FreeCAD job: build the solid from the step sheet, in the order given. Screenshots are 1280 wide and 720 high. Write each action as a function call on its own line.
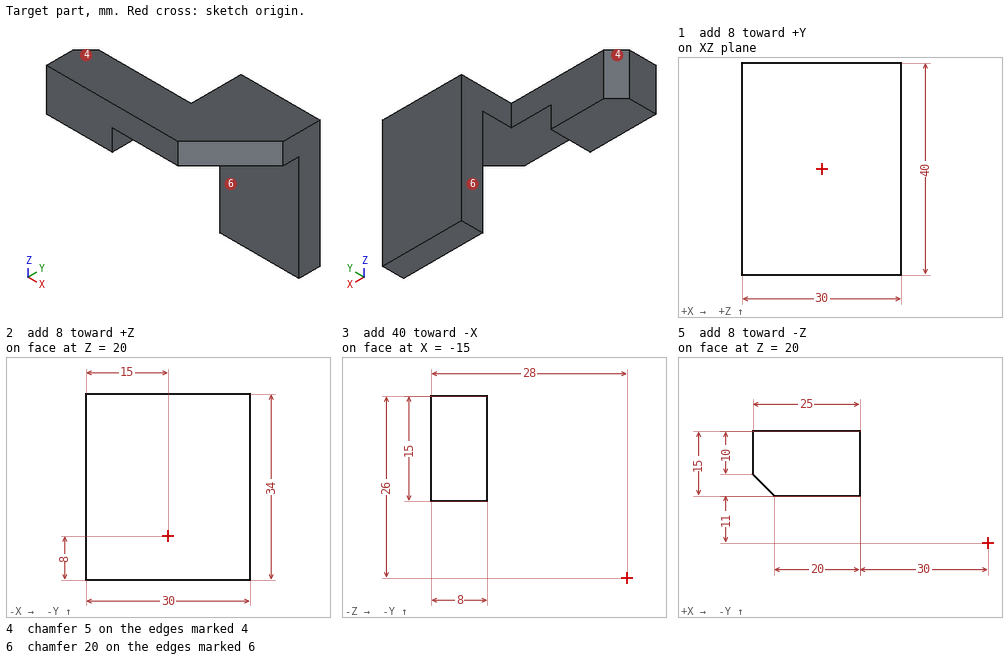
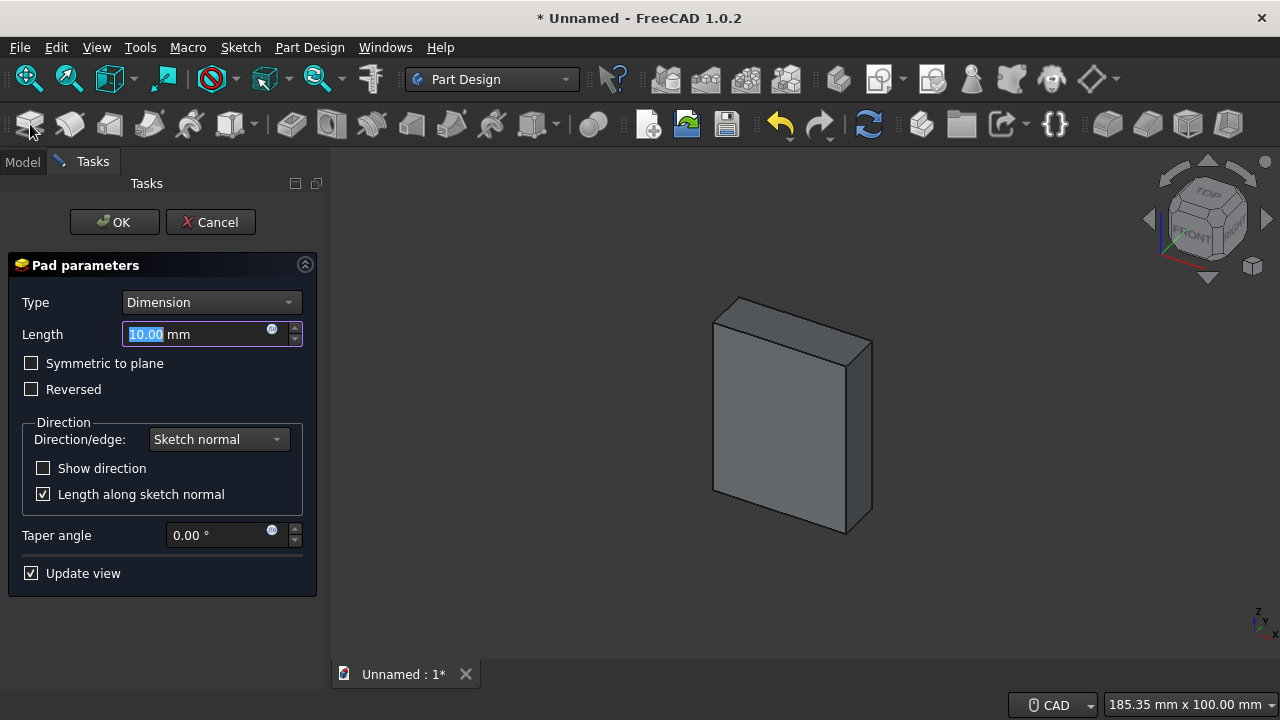
text(8)
key(Tab)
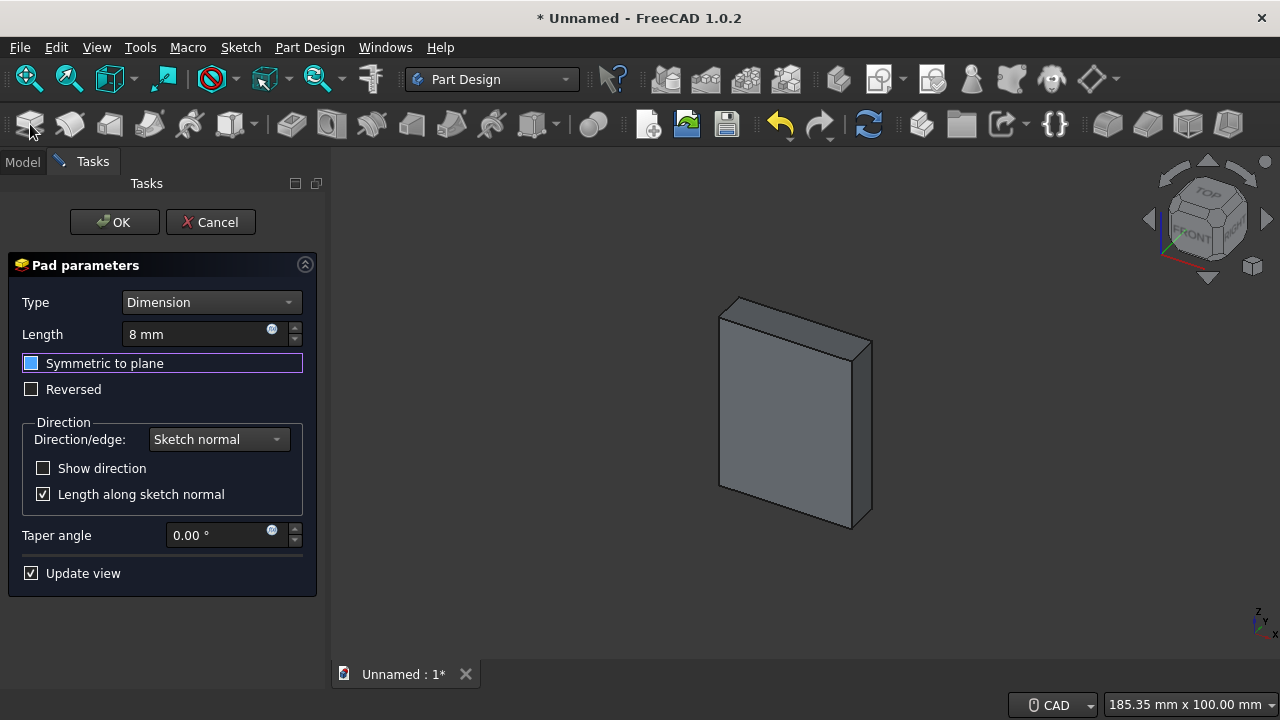
click(30, 389)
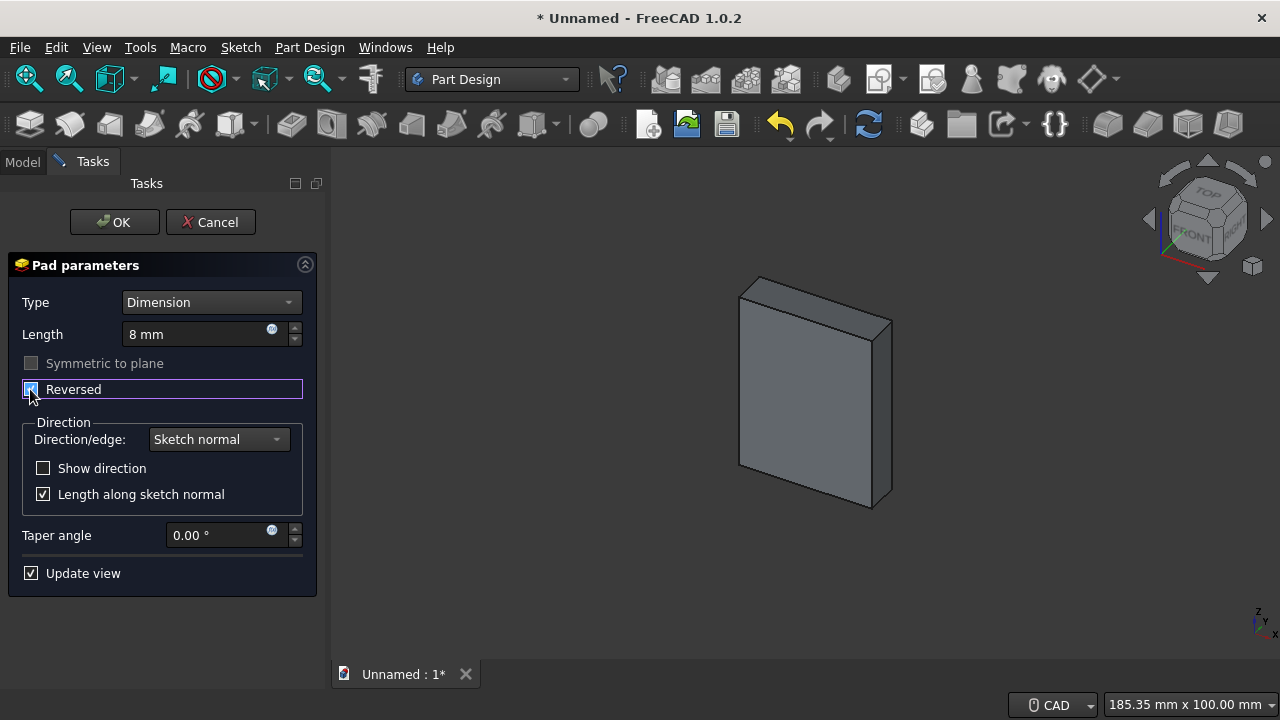
click(115, 222)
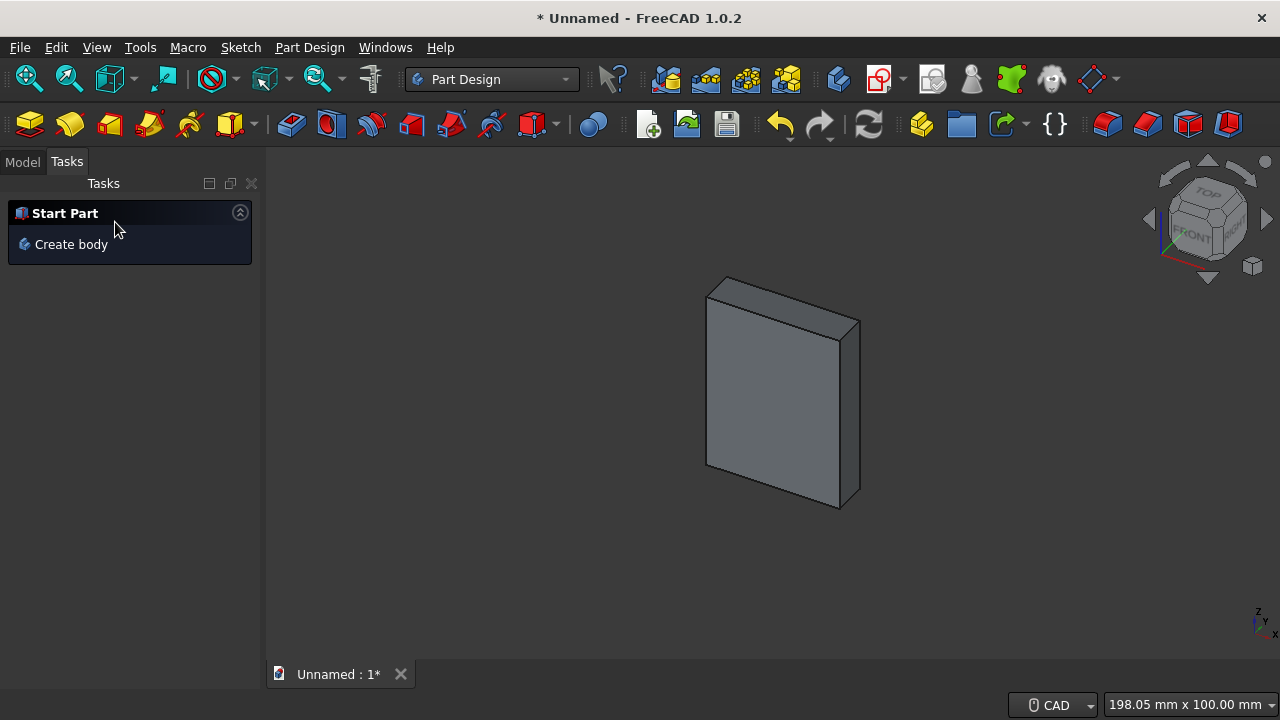
click(821, 321)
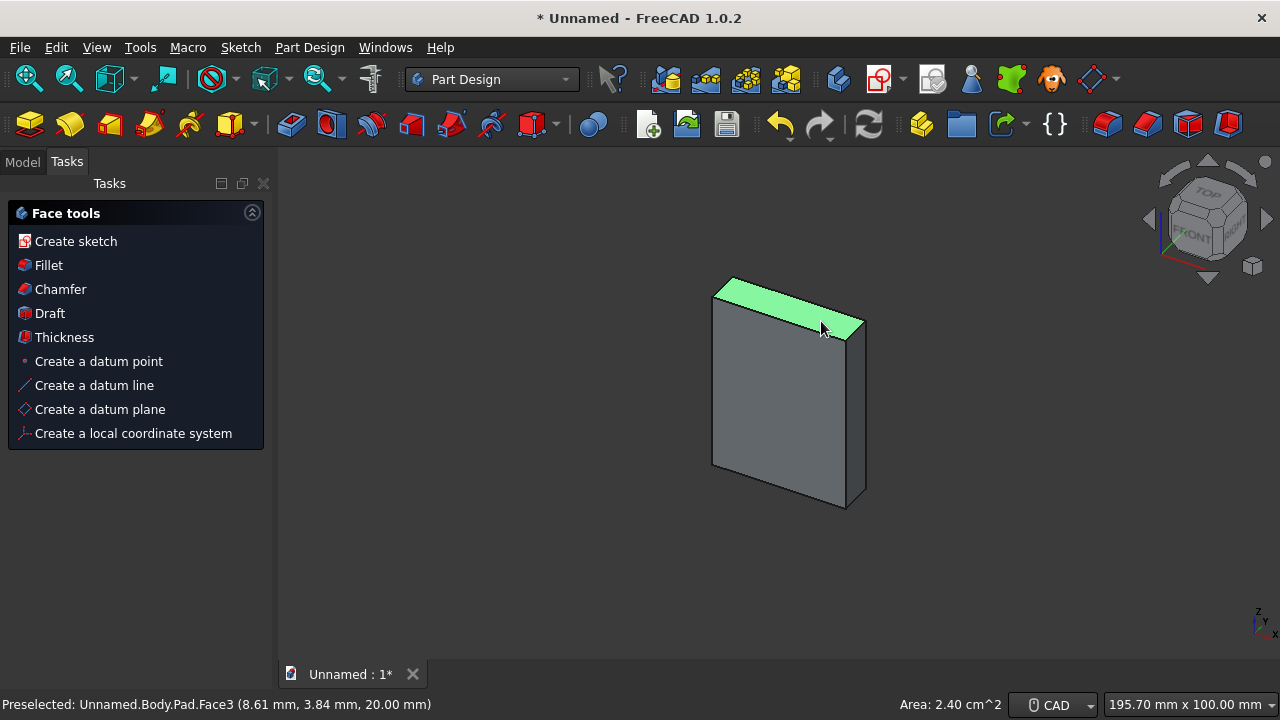
click(880, 80)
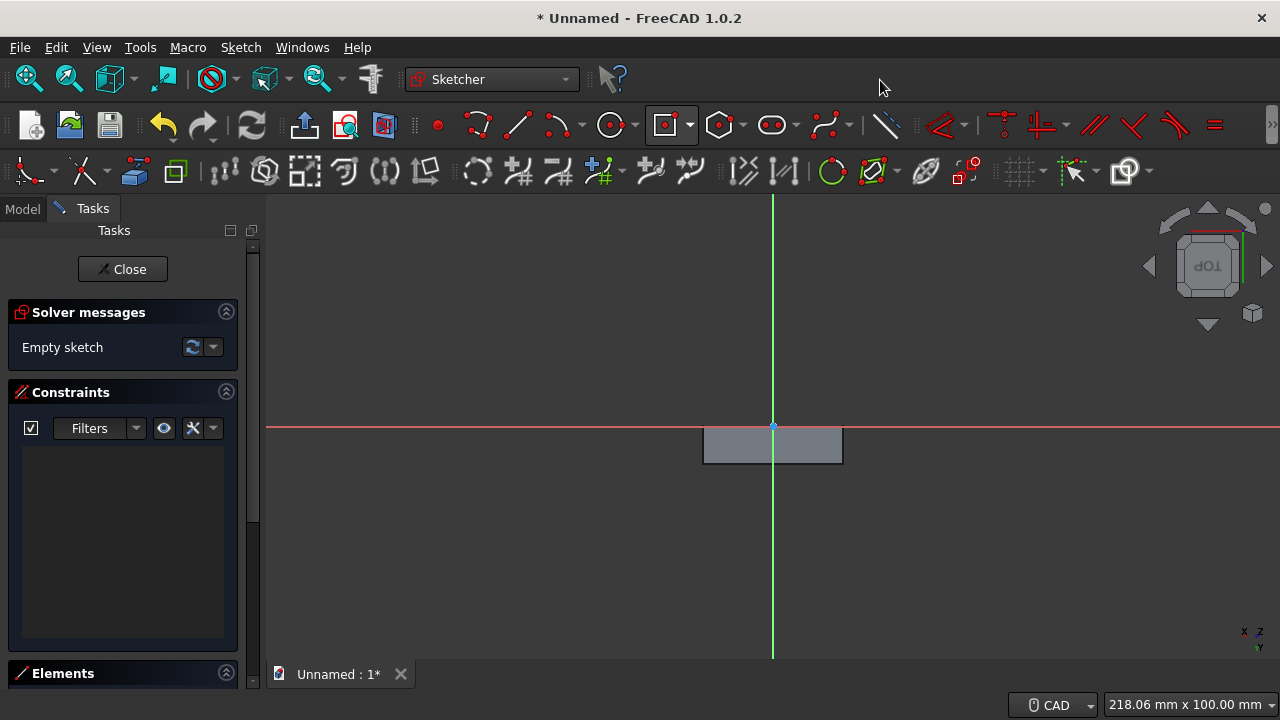
scroll(856, 334, up, 3)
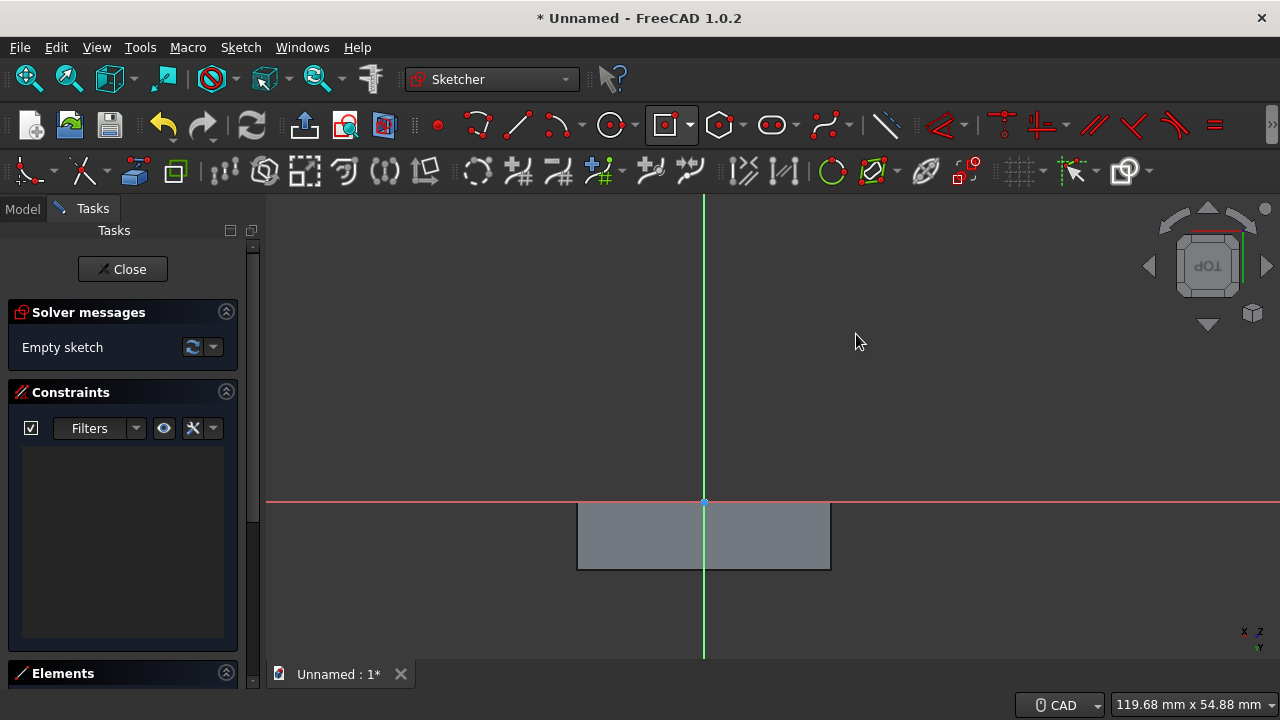
key(g)
key(r)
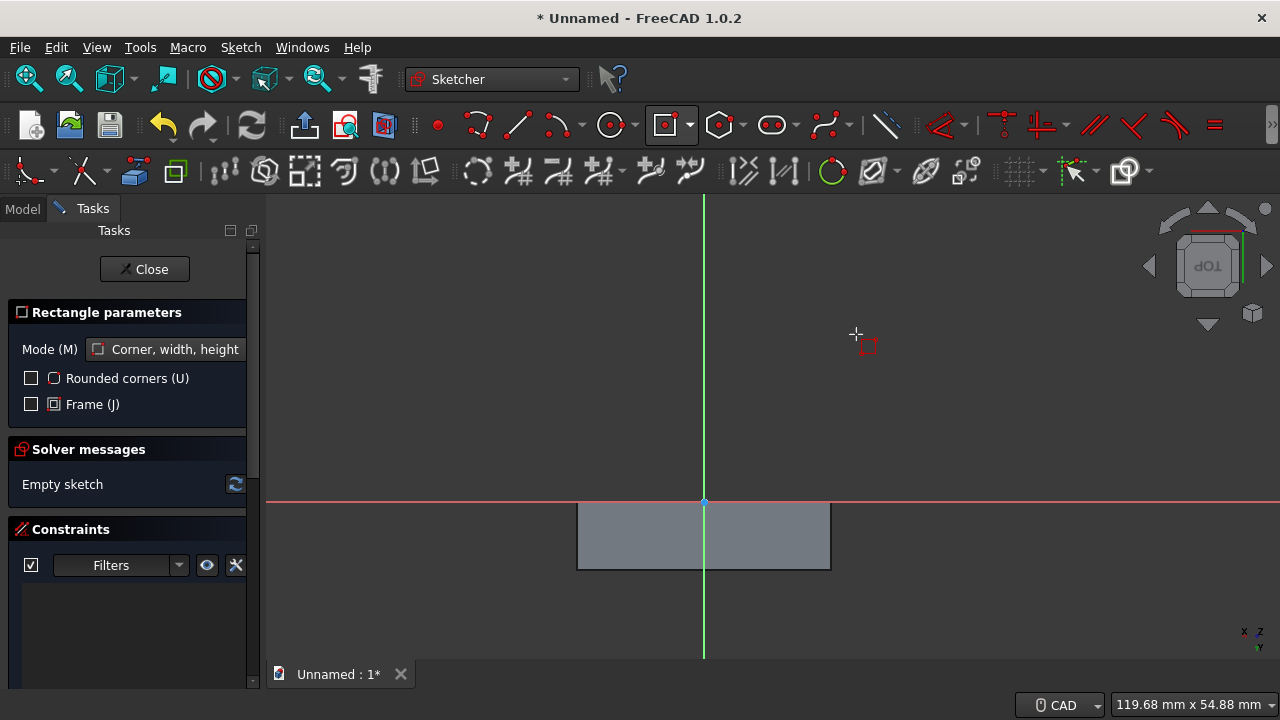
click(577, 282)
move(831, 570)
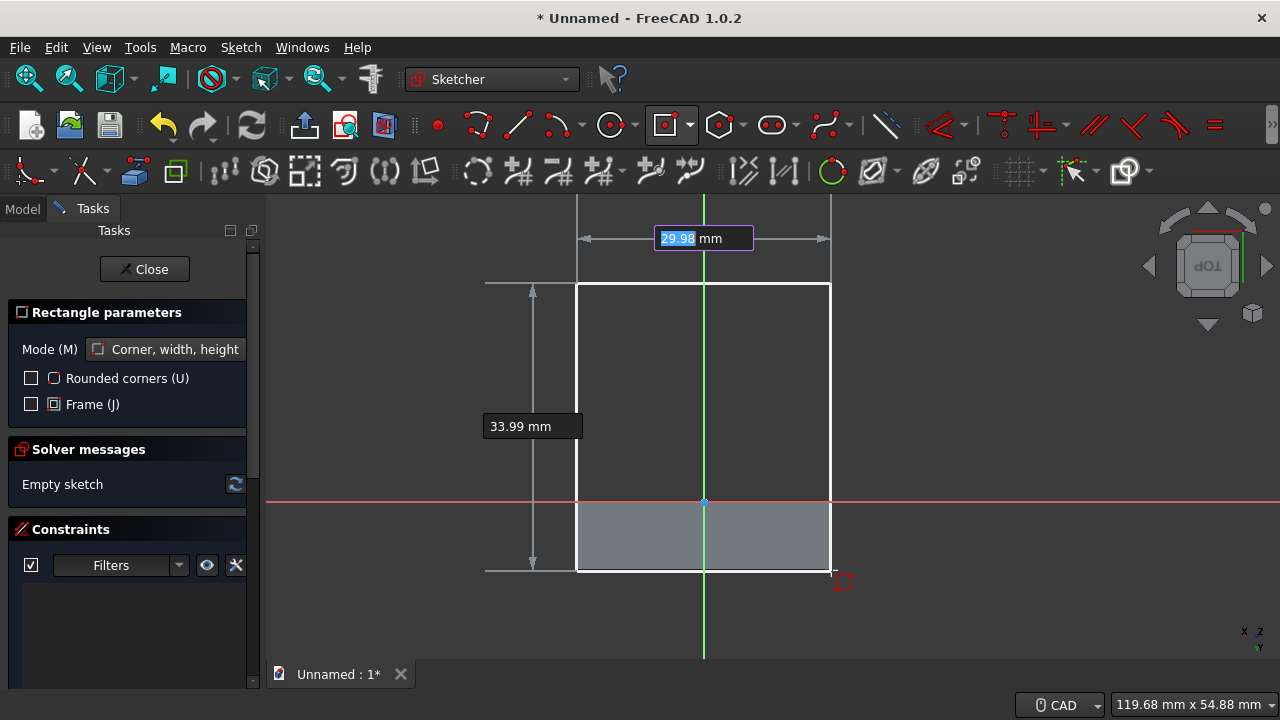
text(30)
key(Tab)
text(34)
key(Return)
key(Escape)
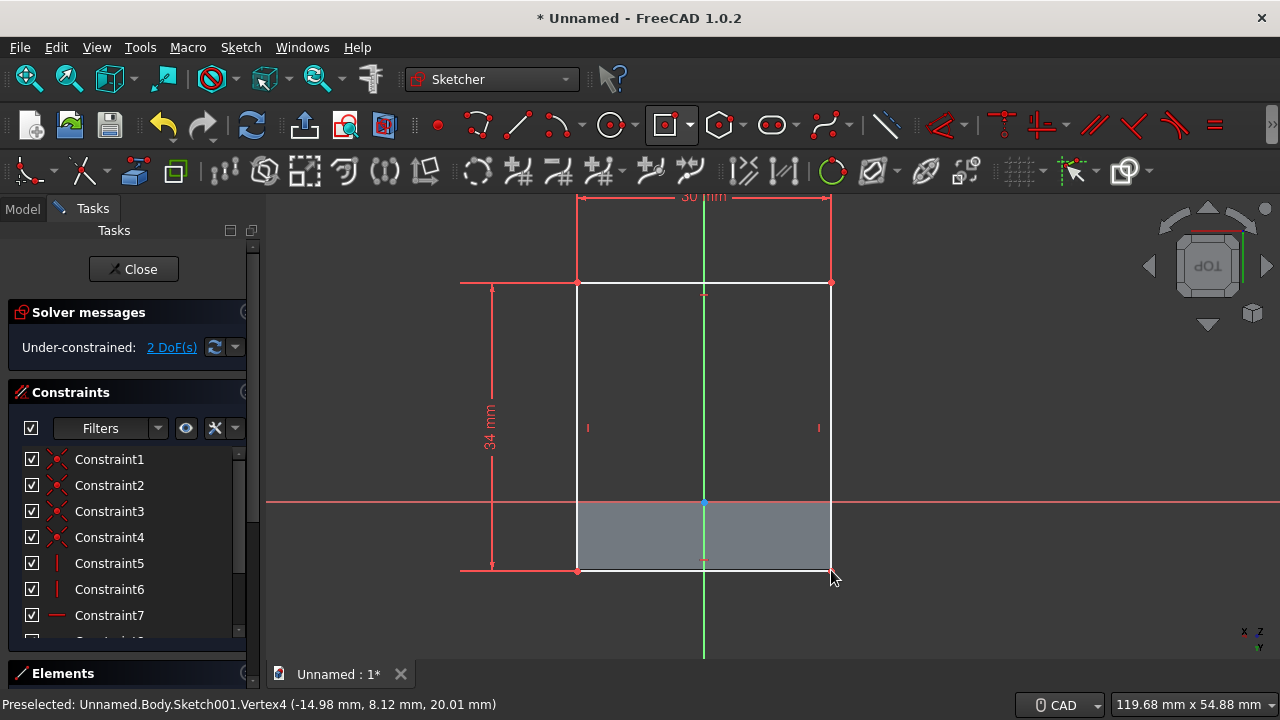
click(940, 126)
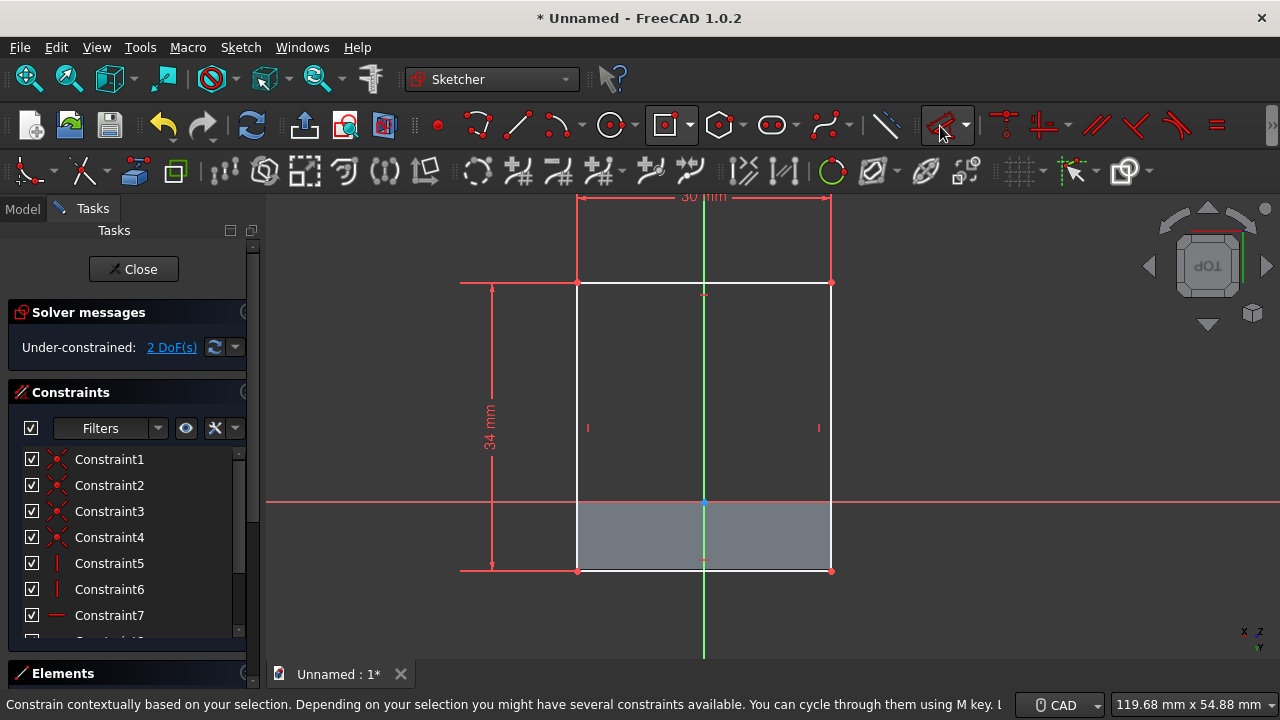
click(577, 571)
click(543, 537)